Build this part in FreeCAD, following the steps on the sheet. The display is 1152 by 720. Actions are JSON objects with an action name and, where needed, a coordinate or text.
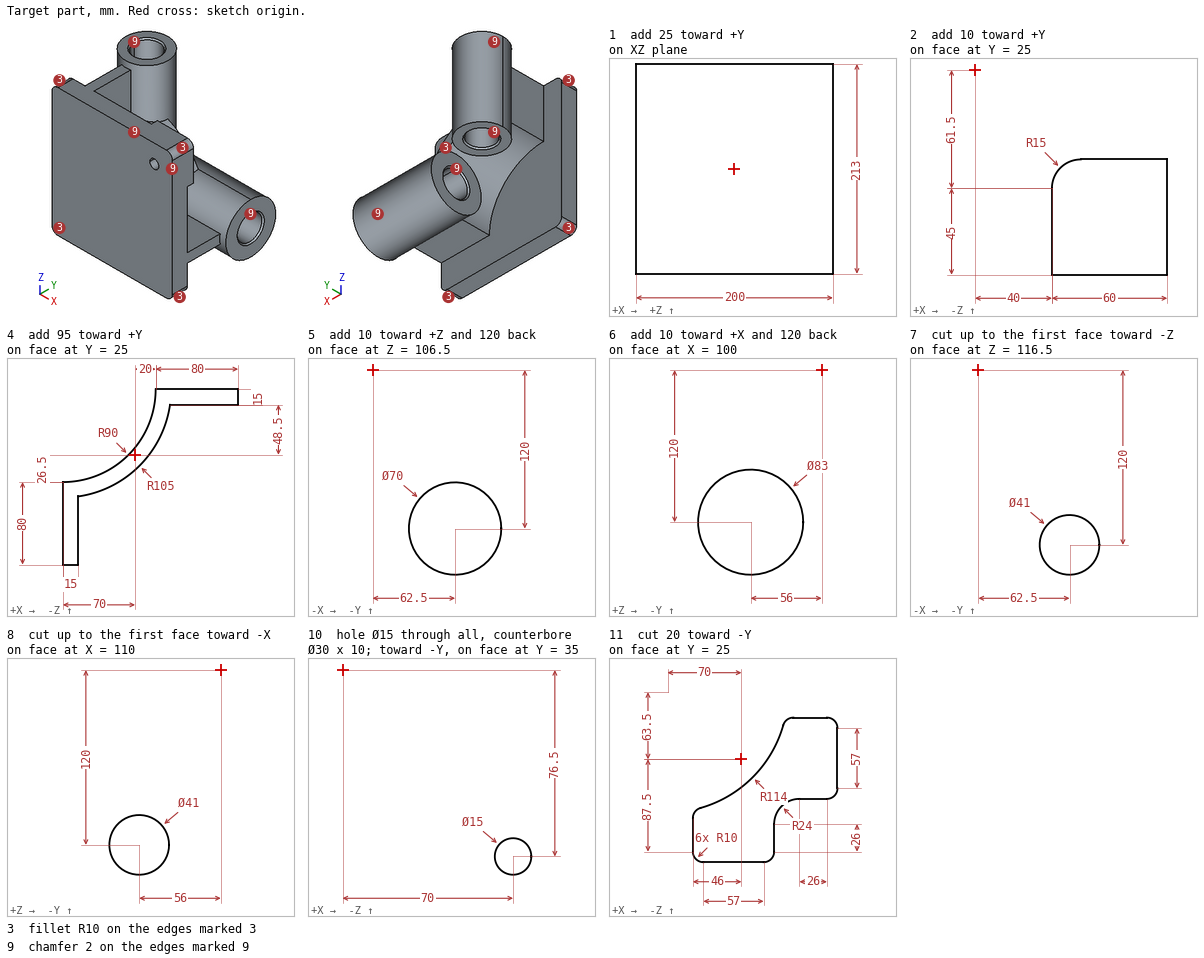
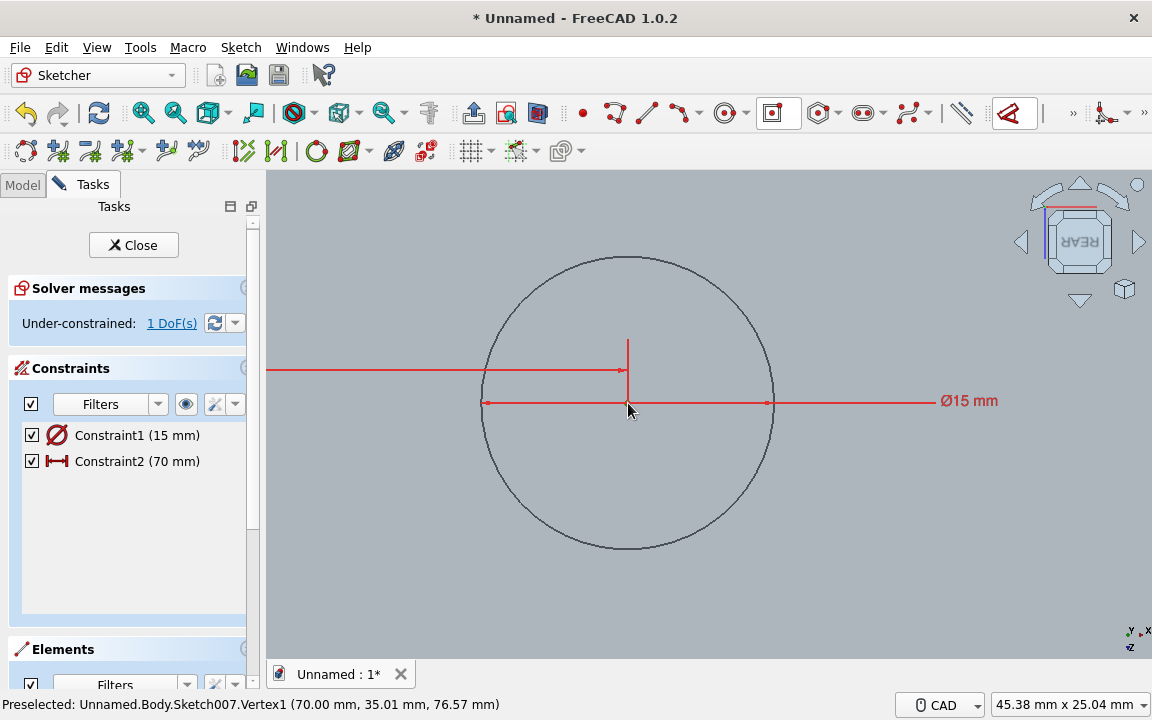
{"action": "left_click", "coordinate": [1032, 114]}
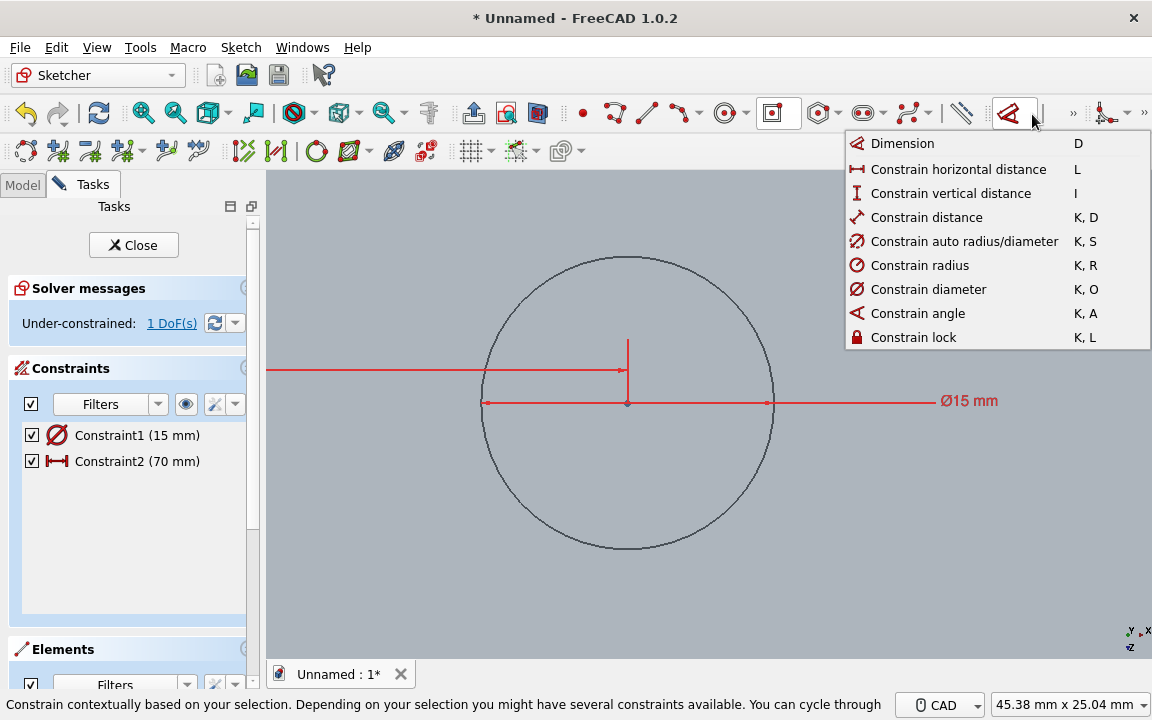
{"action": "left_click", "coordinate": [998, 193]}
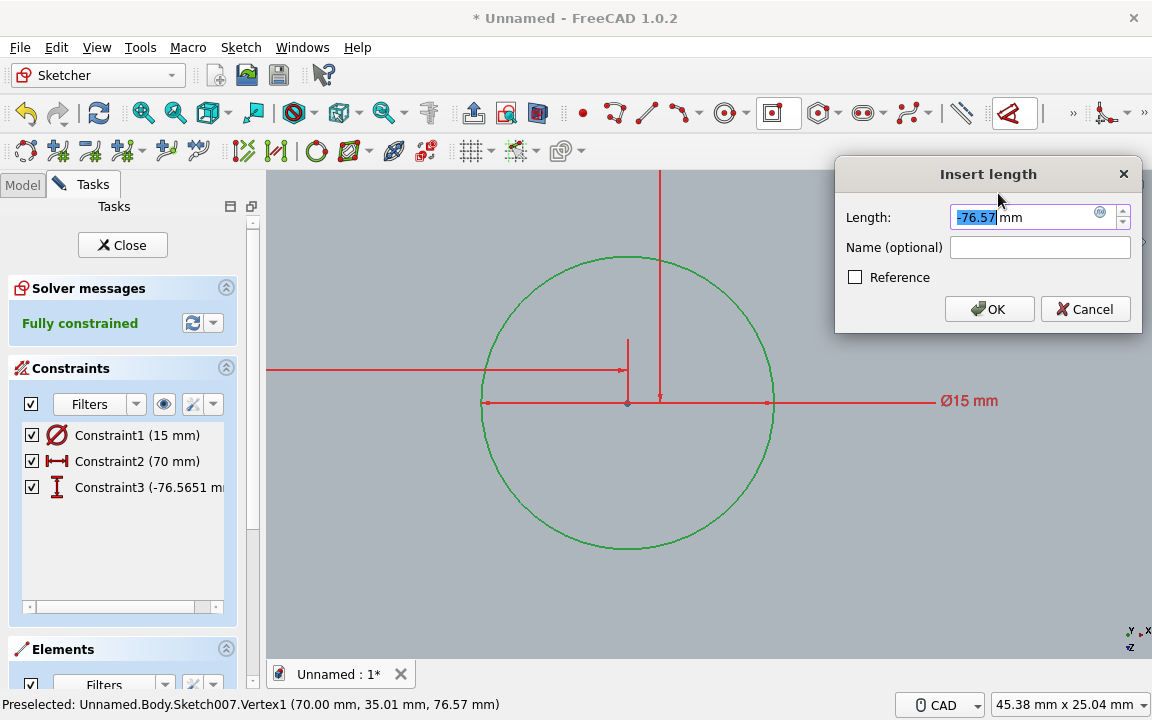
{"action": "type", "text": "-76.5"}
{"action": "key", "text": "Return"}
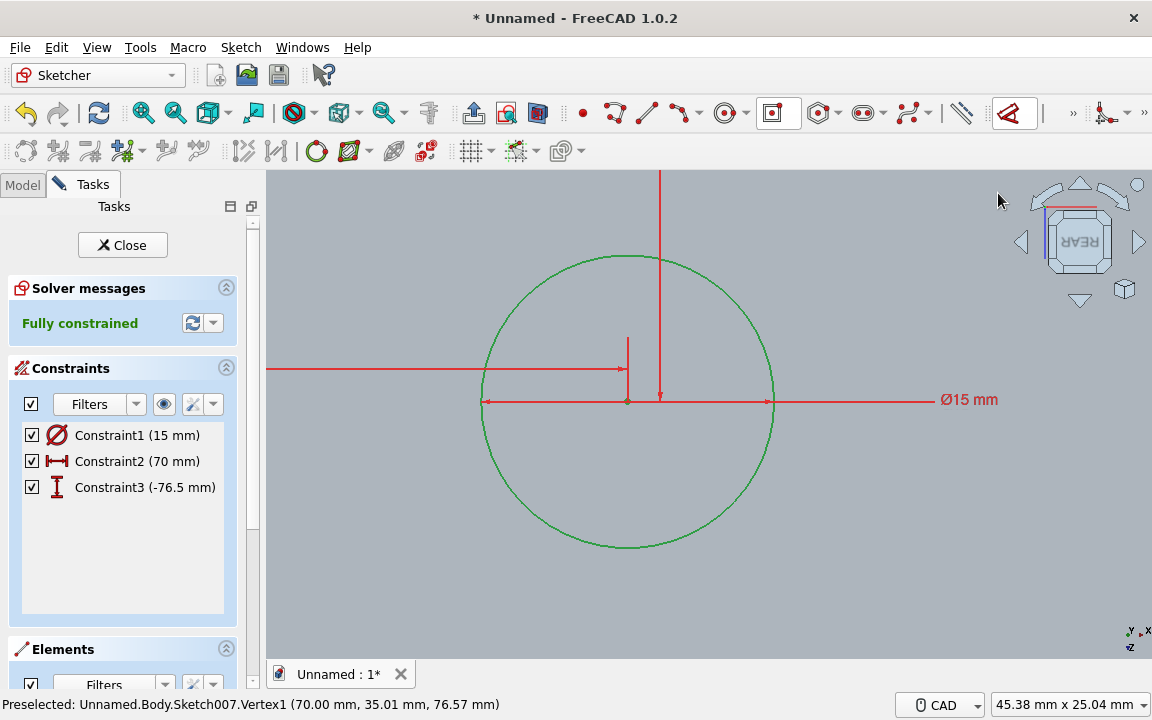
{"action": "left_click", "coordinate": [123, 245]}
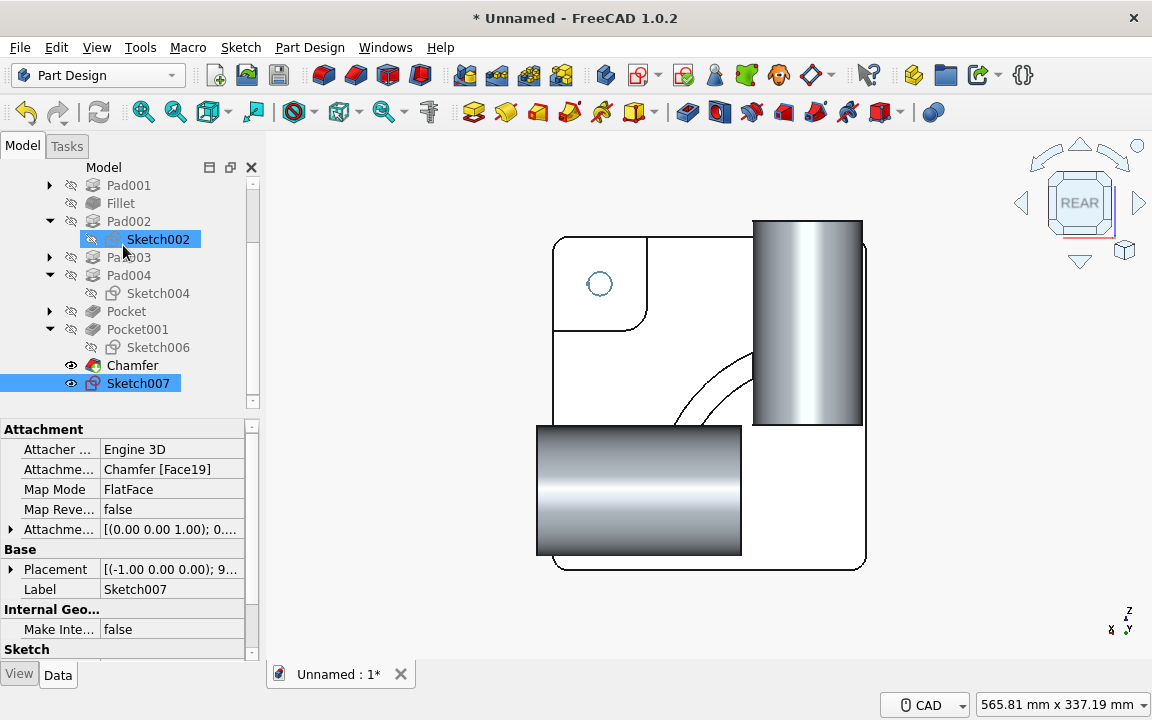
{"action": "left_click", "coordinate": [720, 112]}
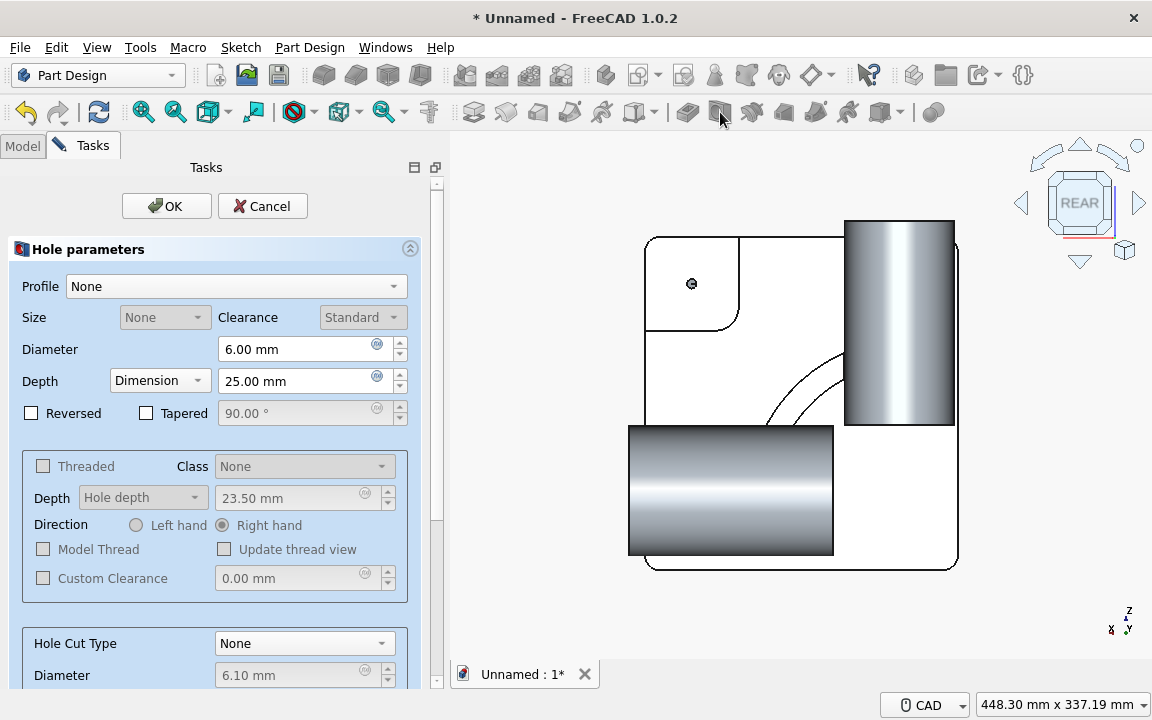
{"action": "triple_click", "coordinate": [305, 349]}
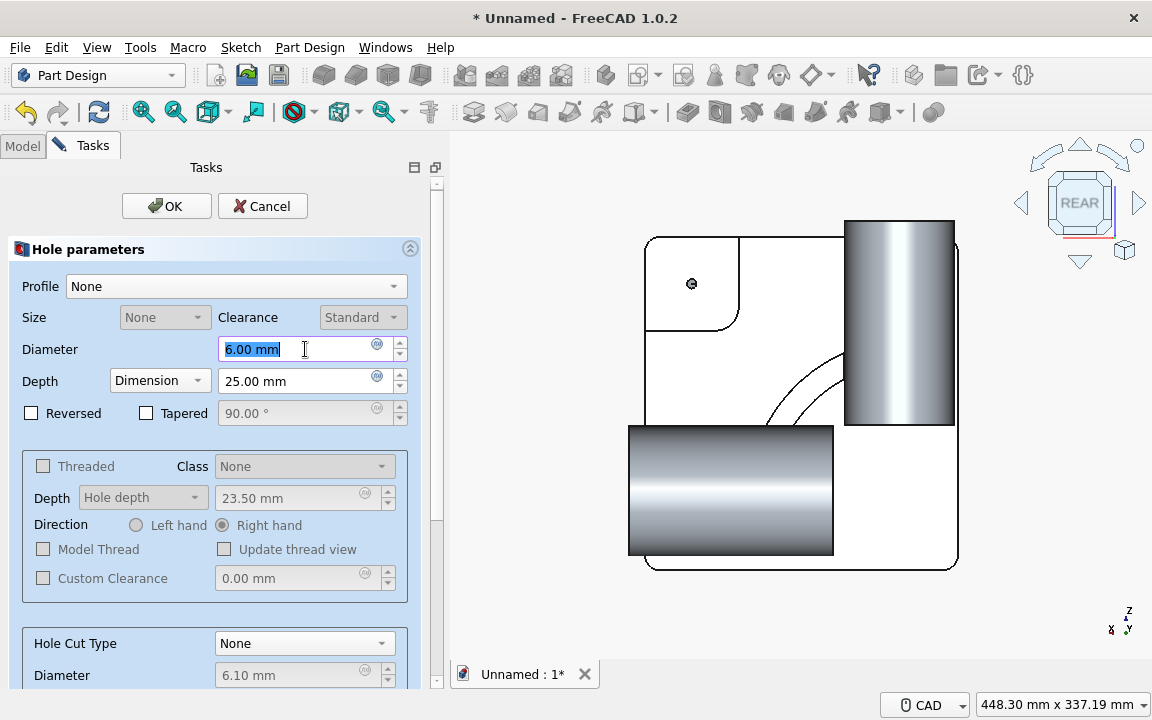
{"action": "type", "text": "15"}
{"action": "key", "text": "Tab"}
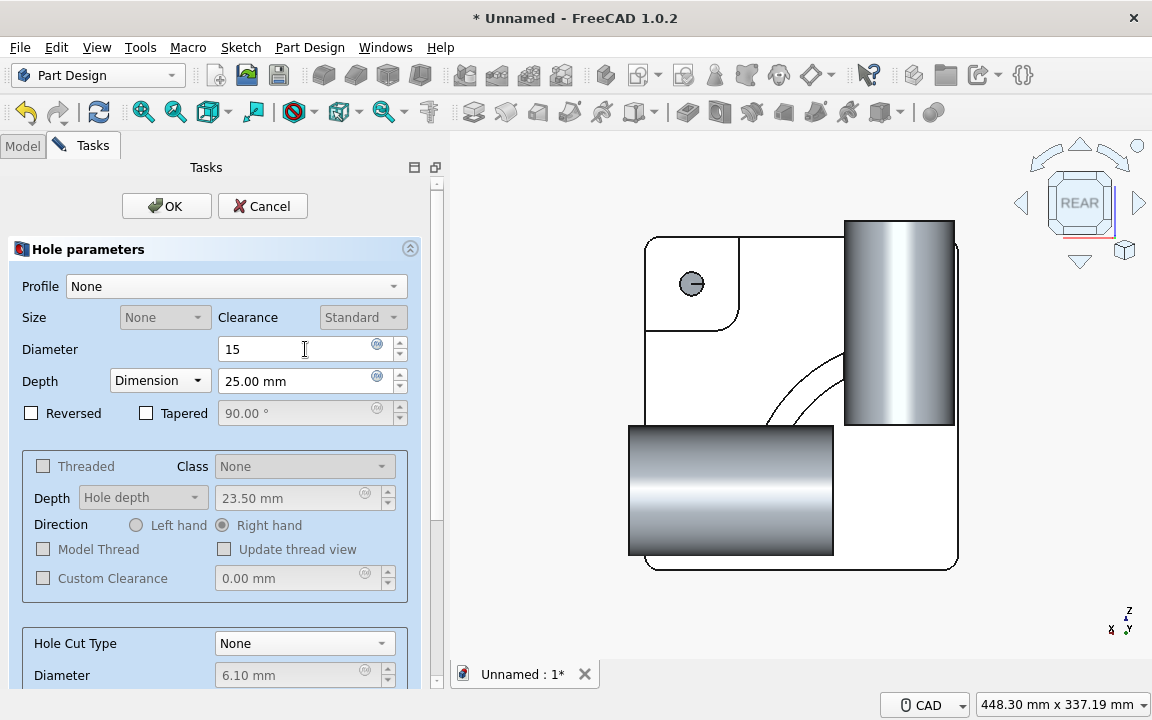
{"action": "left_click", "coordinate": [161, 380]}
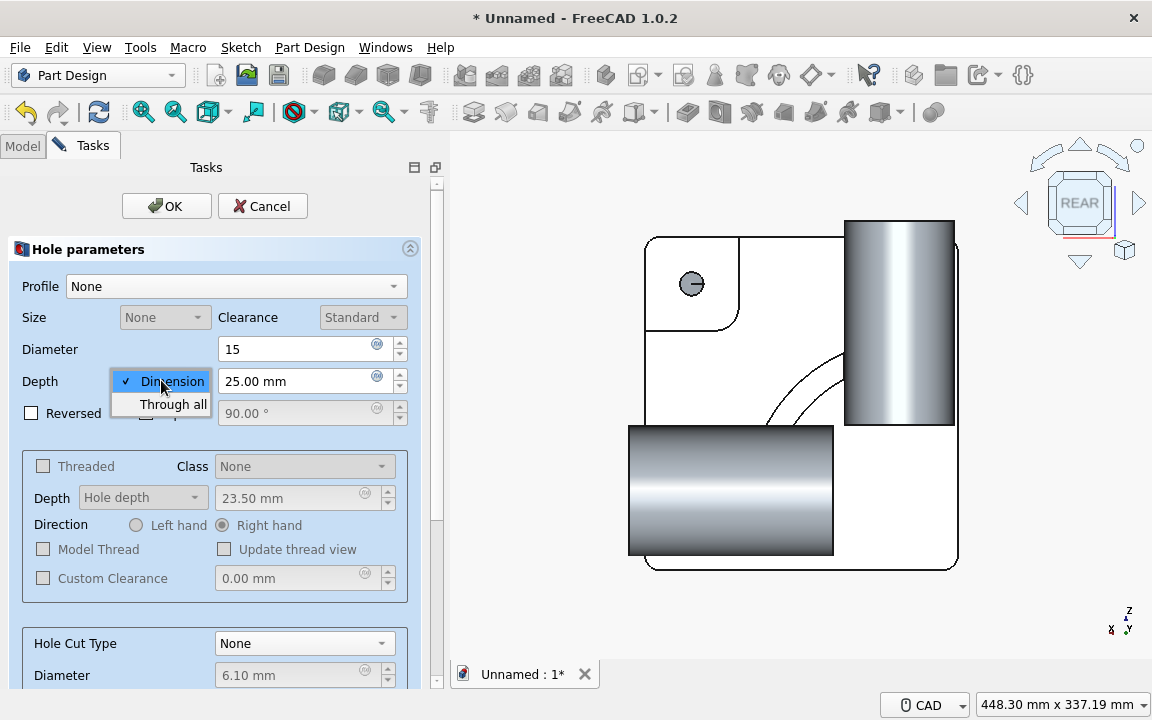
{"action": "left_click", "coordinate": [160, 404]}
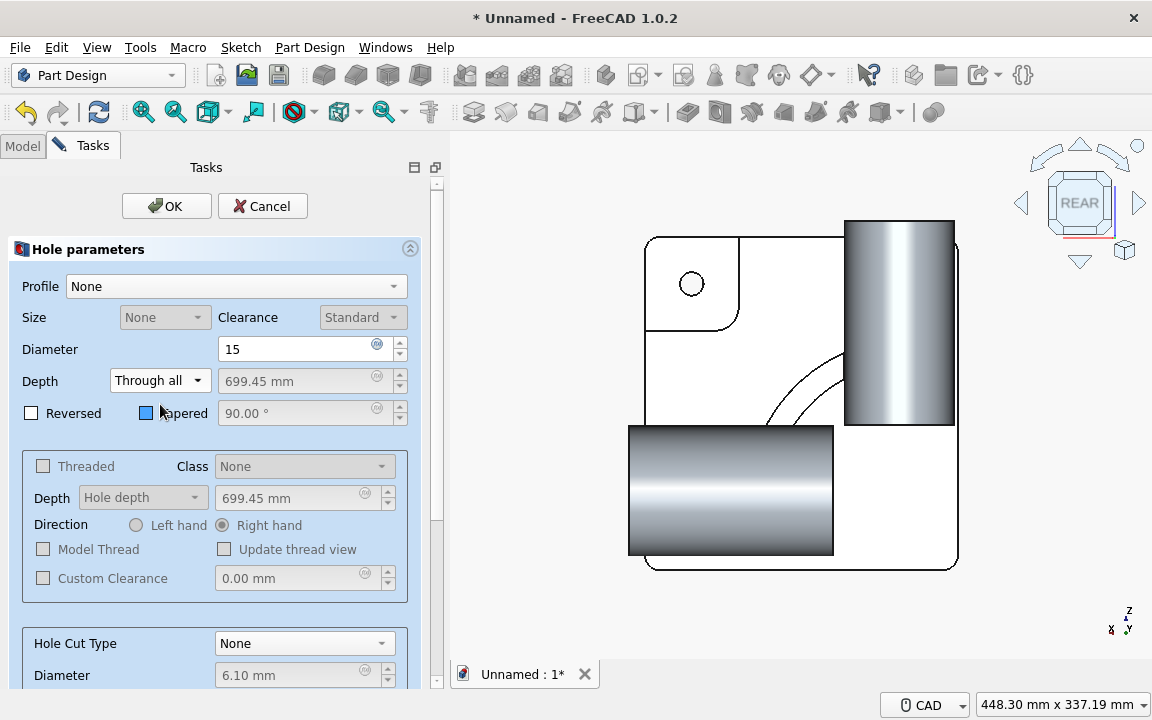
{"action": "left_click", "coordinate": [306, 644]}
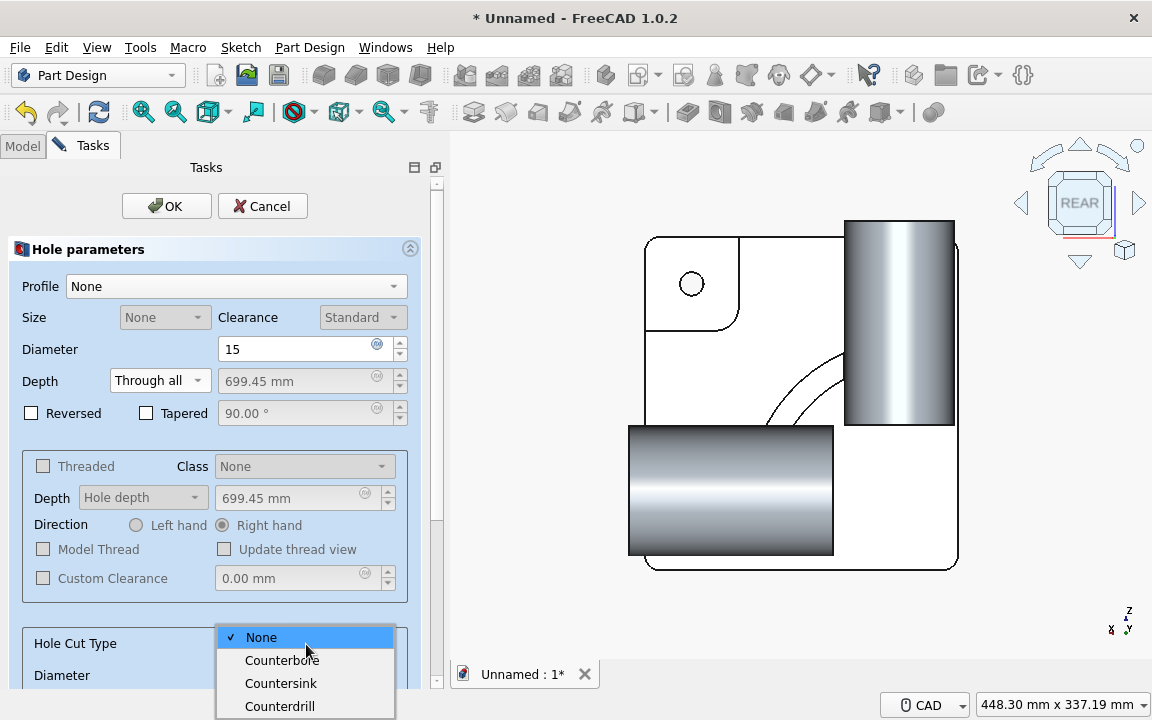
{"action": "left_click", "coordinate": [304, 660]}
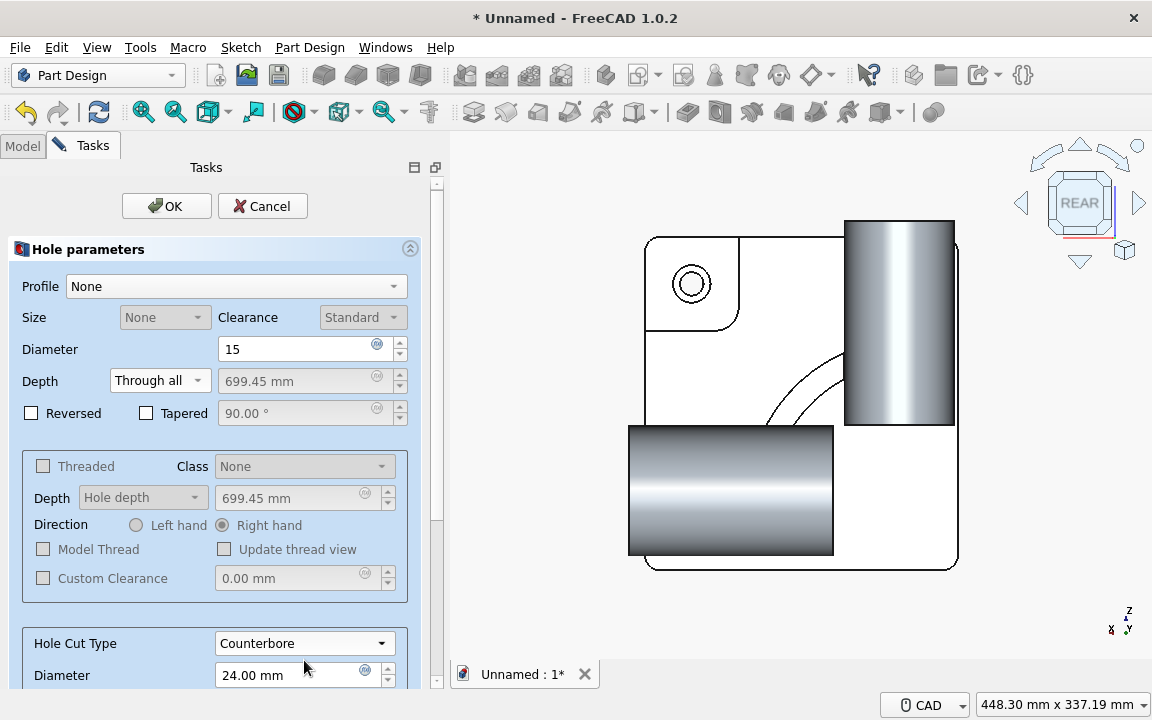
{"action": "triple_click", "coordinate": [298, 675]}